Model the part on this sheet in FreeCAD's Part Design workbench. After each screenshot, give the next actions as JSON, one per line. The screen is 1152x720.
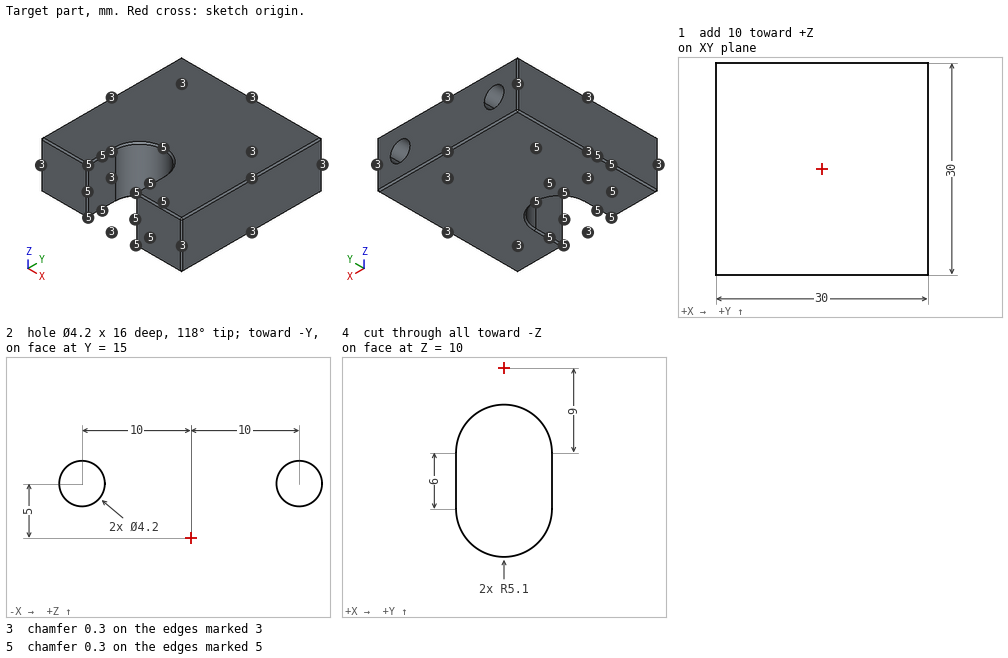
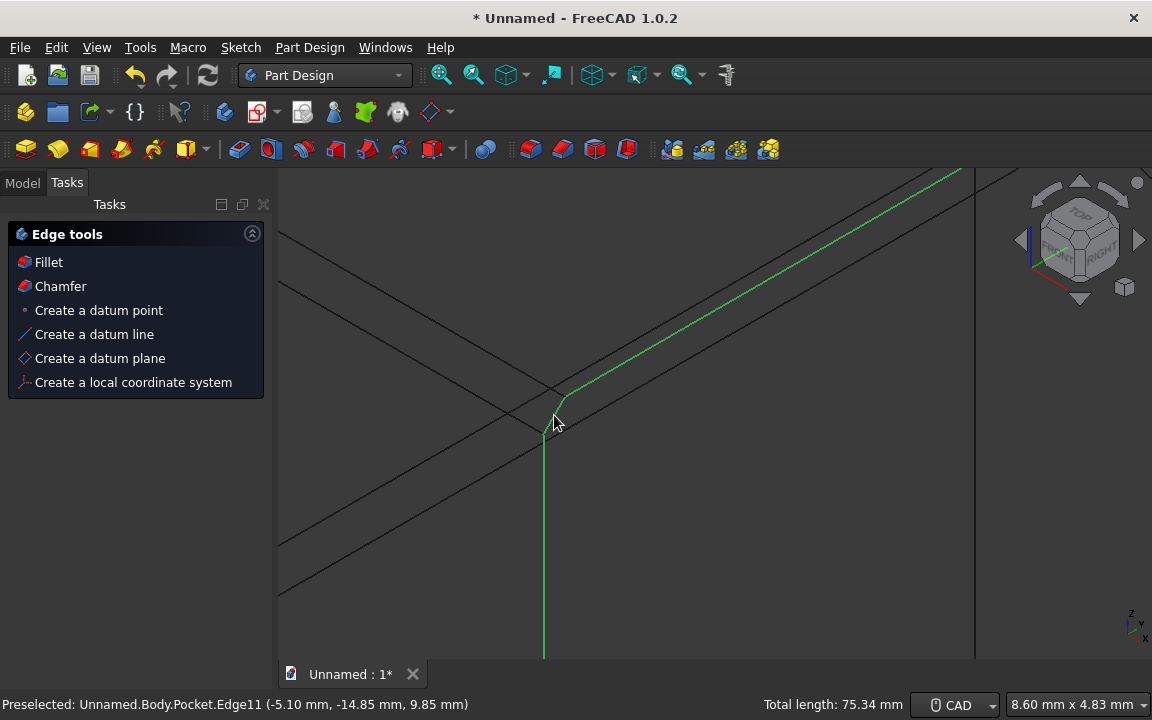
{"action": "key", "text": "v 1"}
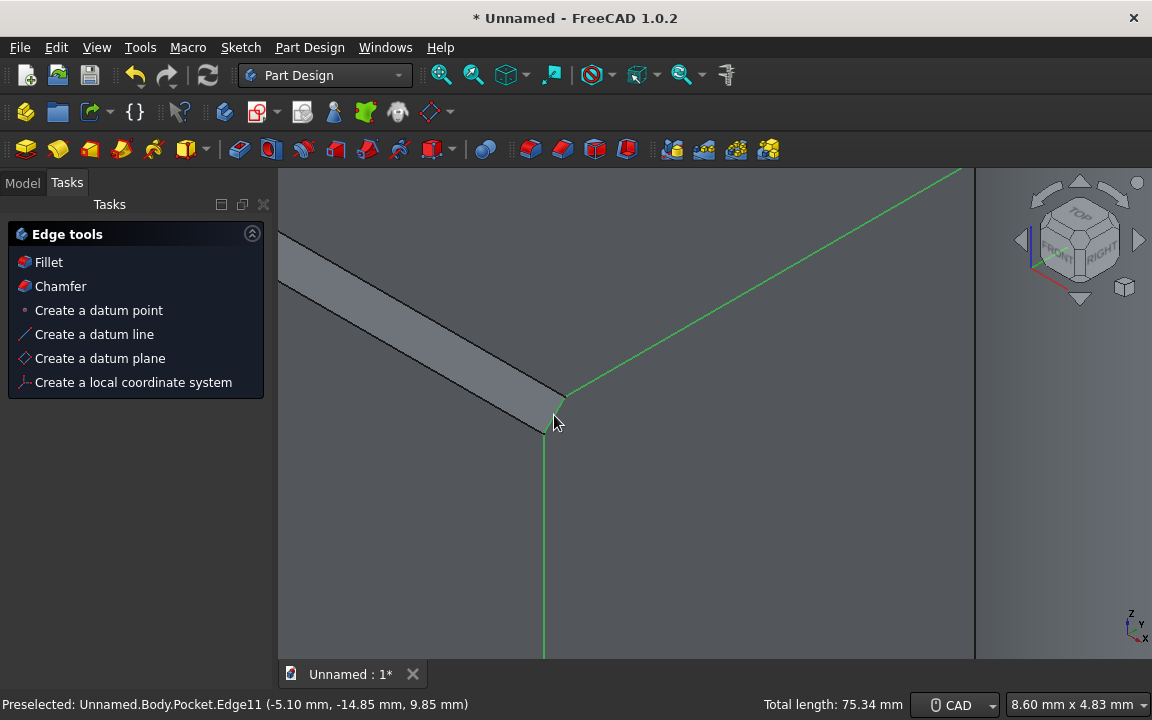
{"action": "left_click", "coordinate": [564, 150]}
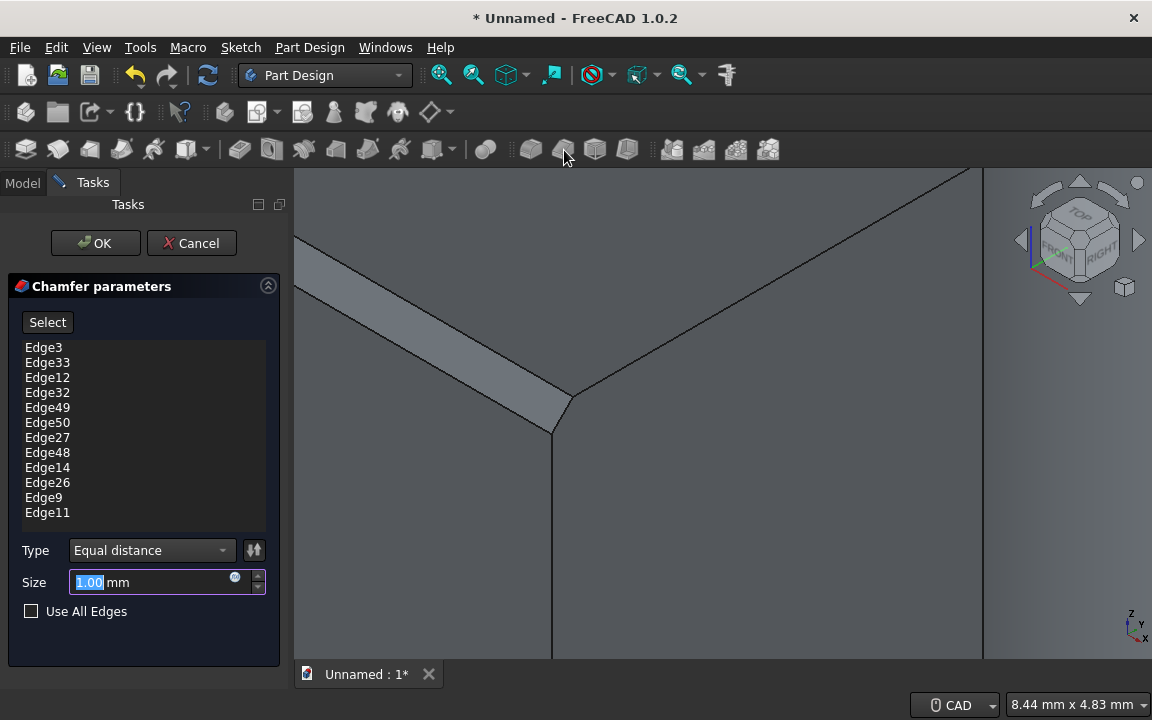
{"action": "type", "text": "0.3"}
{"action": "key", "text": "Tab"}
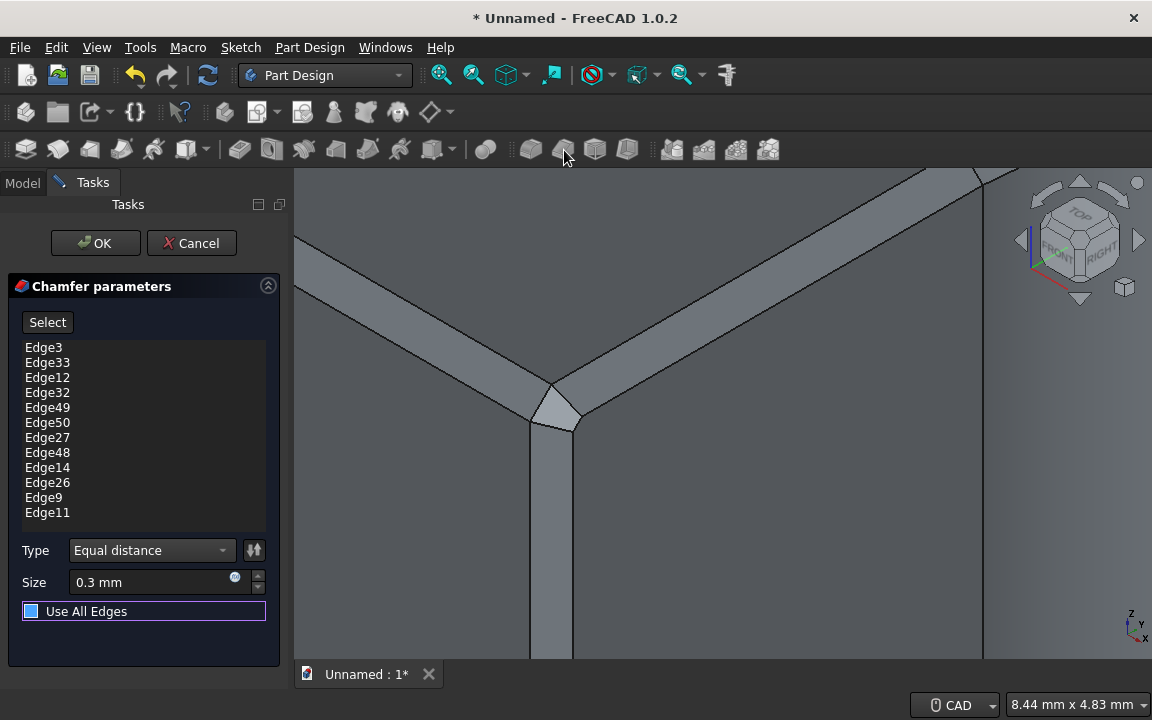
{"action": "left_click", "coordinate": [96, 243]}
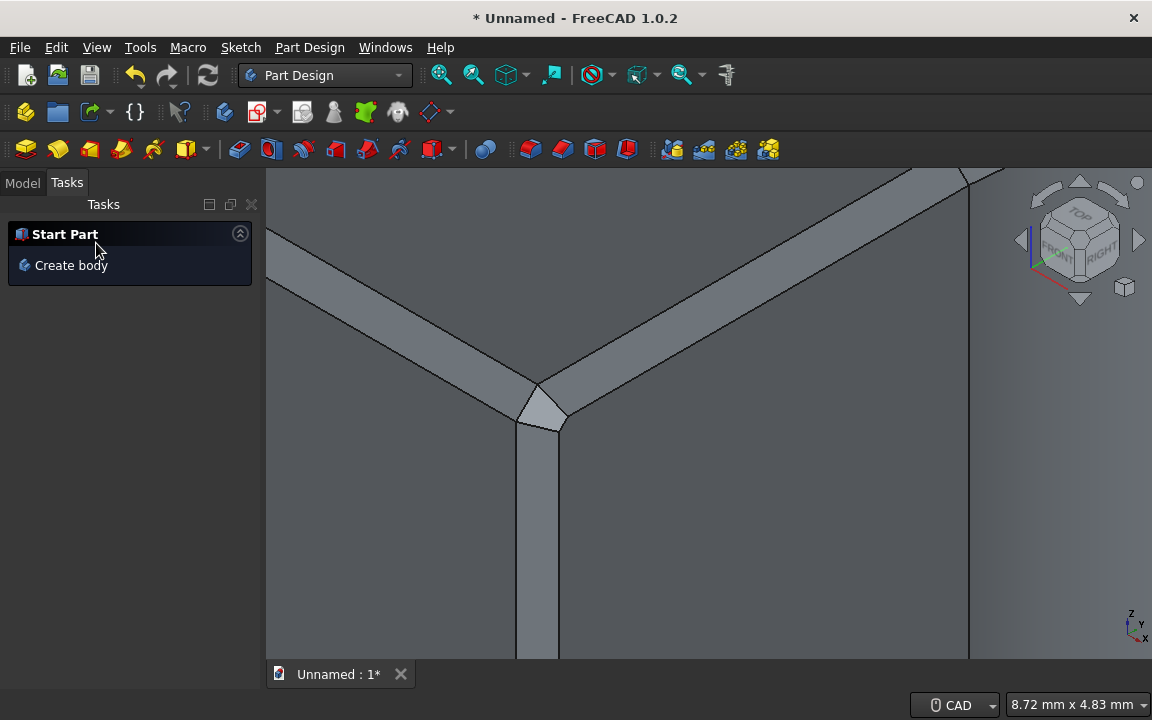
{"action": "left_click", "coordinate": [442, 76]}